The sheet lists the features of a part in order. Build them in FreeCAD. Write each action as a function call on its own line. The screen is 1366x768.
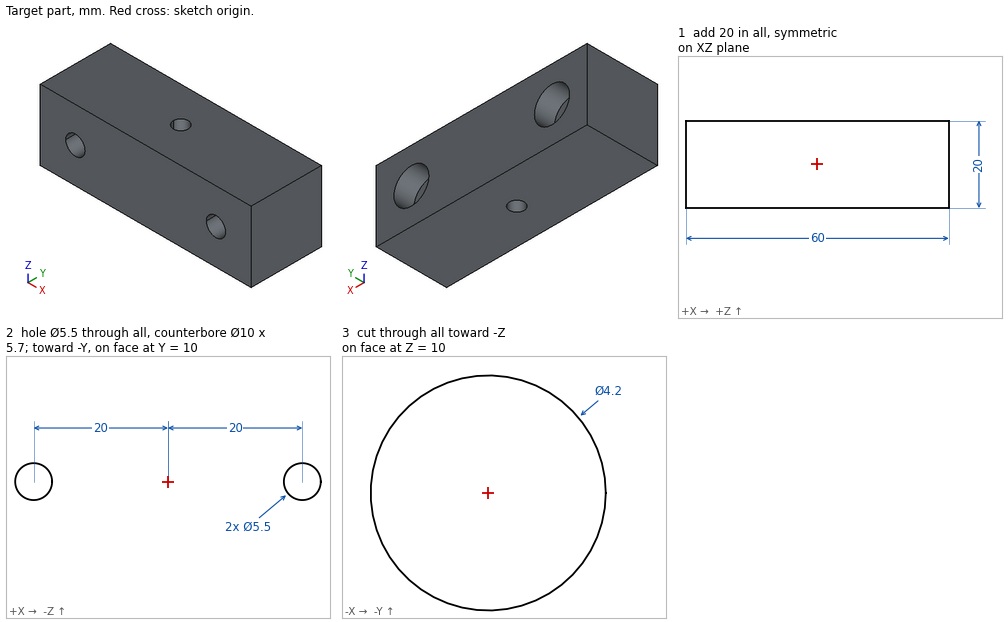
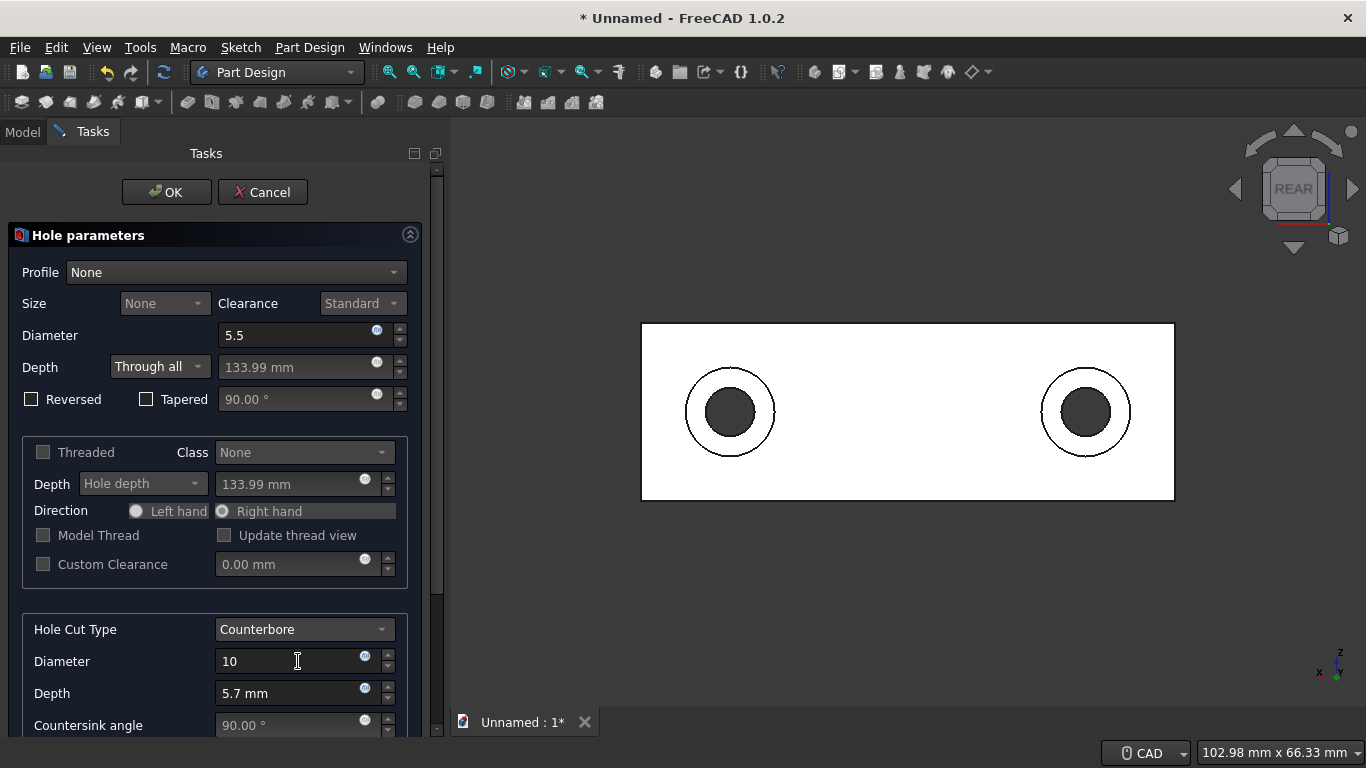
click(167, 192)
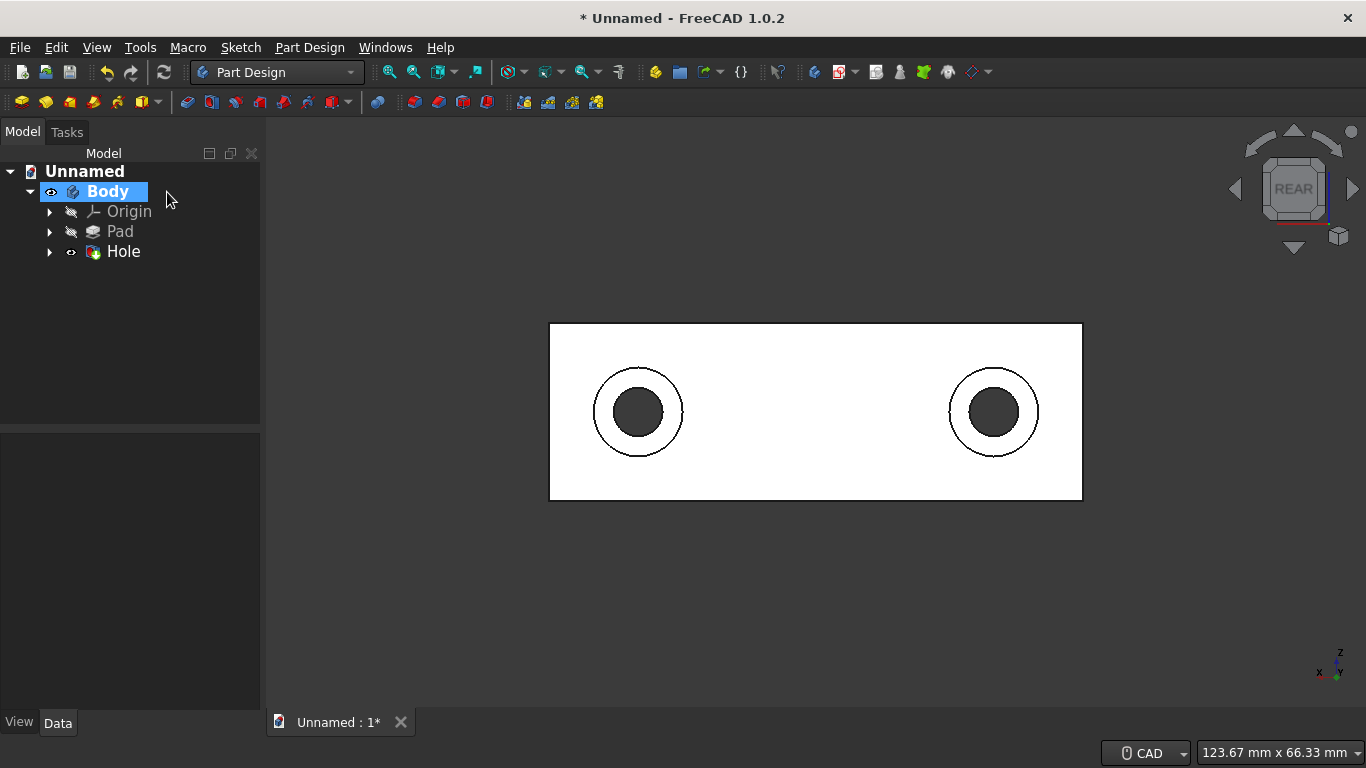
key(0)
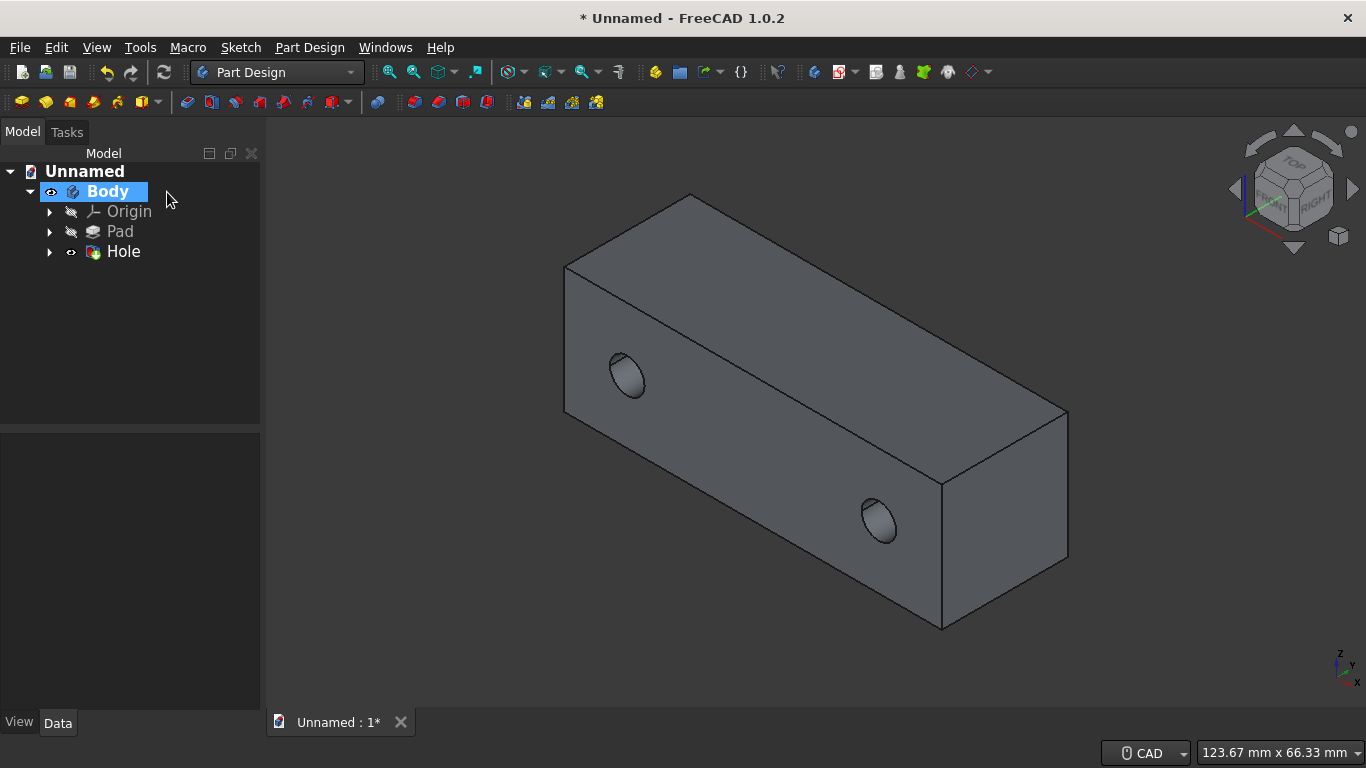
click(924, 401)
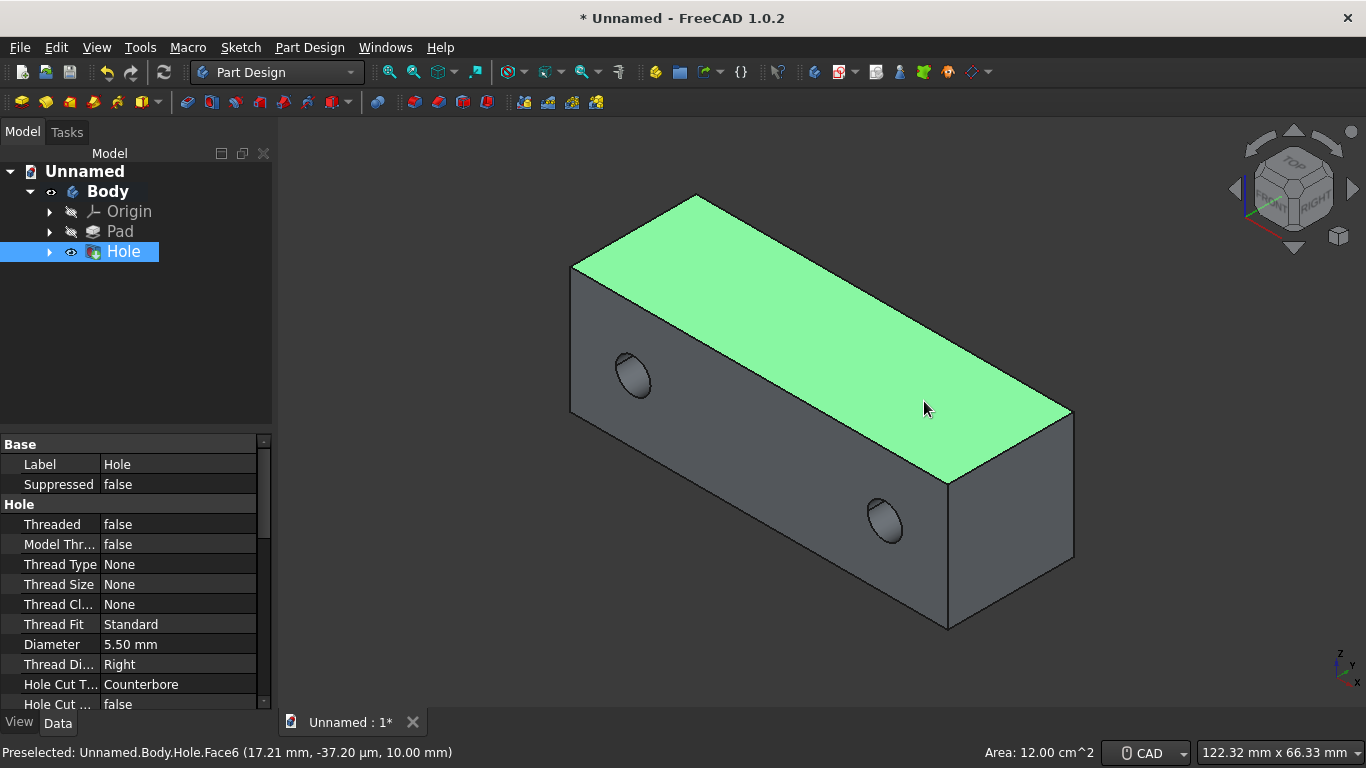
click(840, 72)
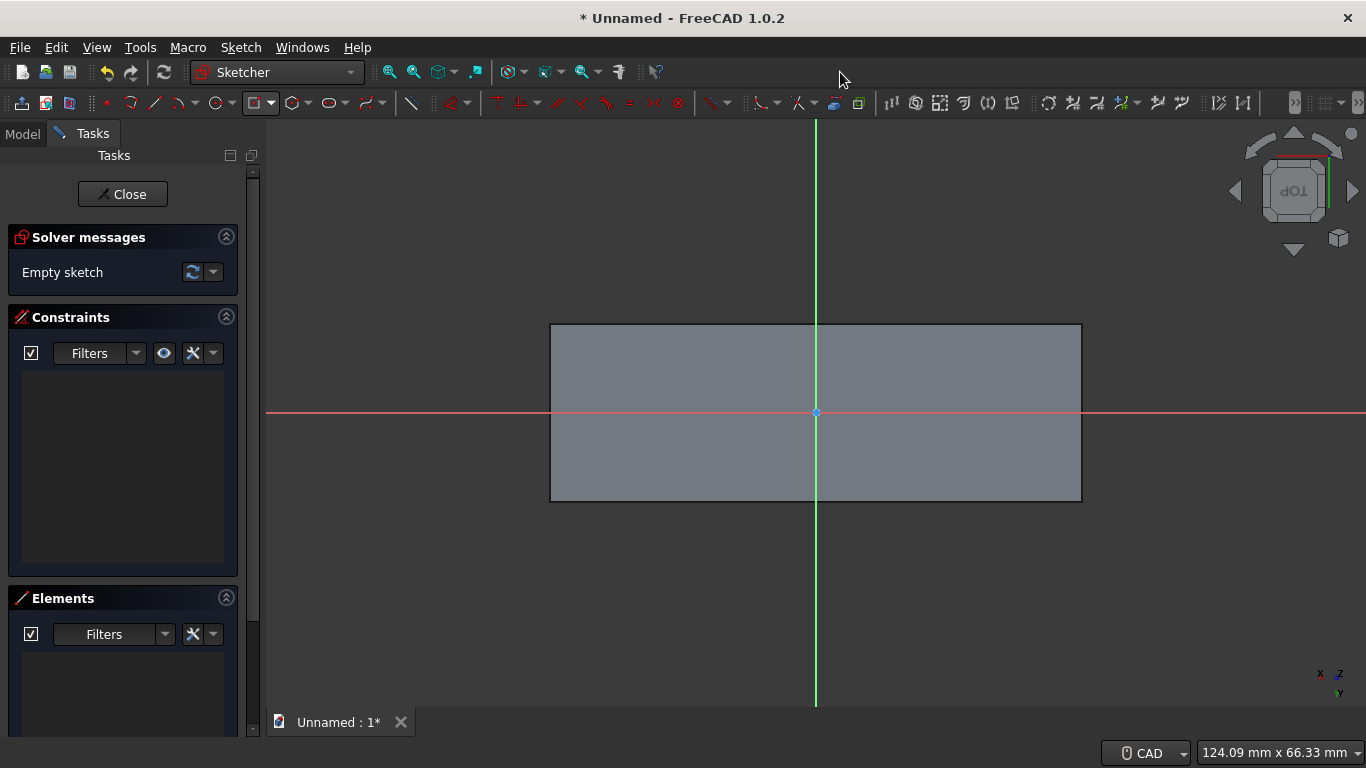
scroll(823, 413, up, 12)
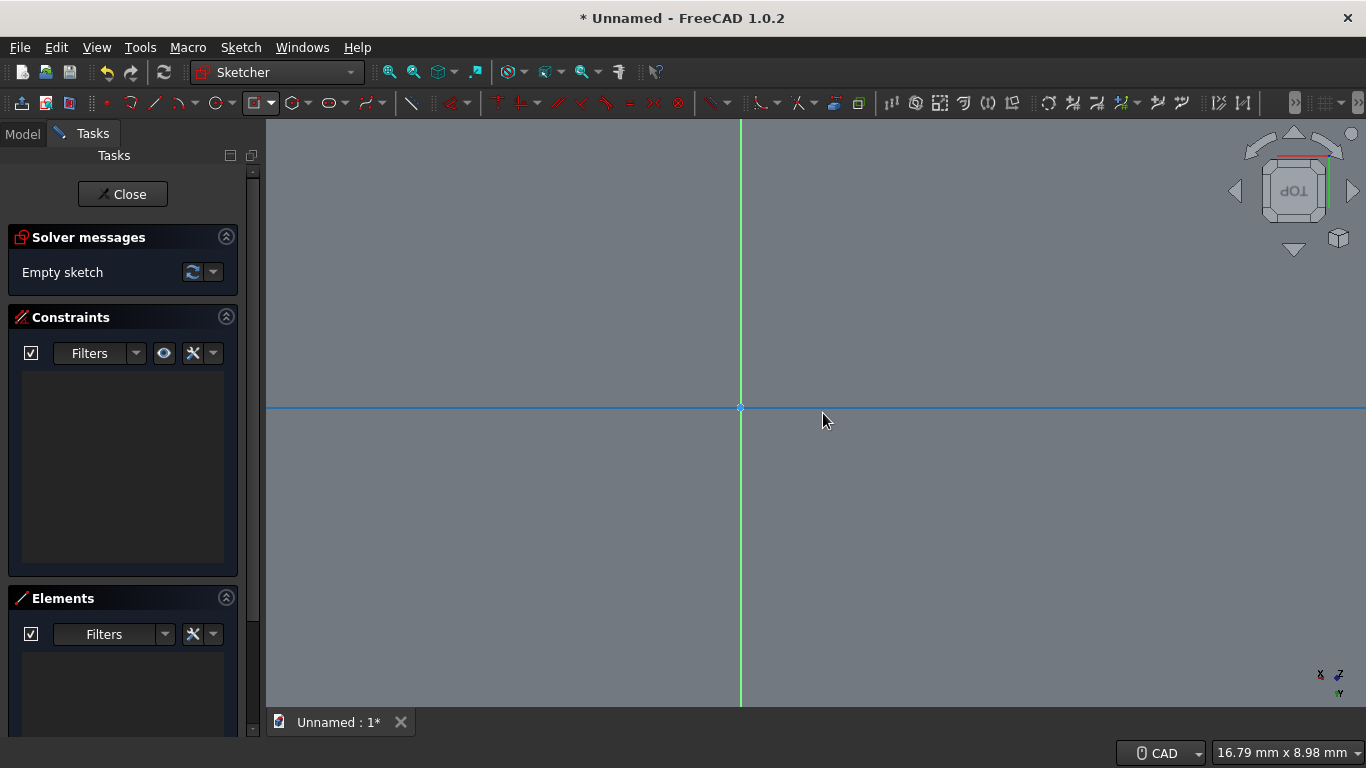
key(g)
key(c)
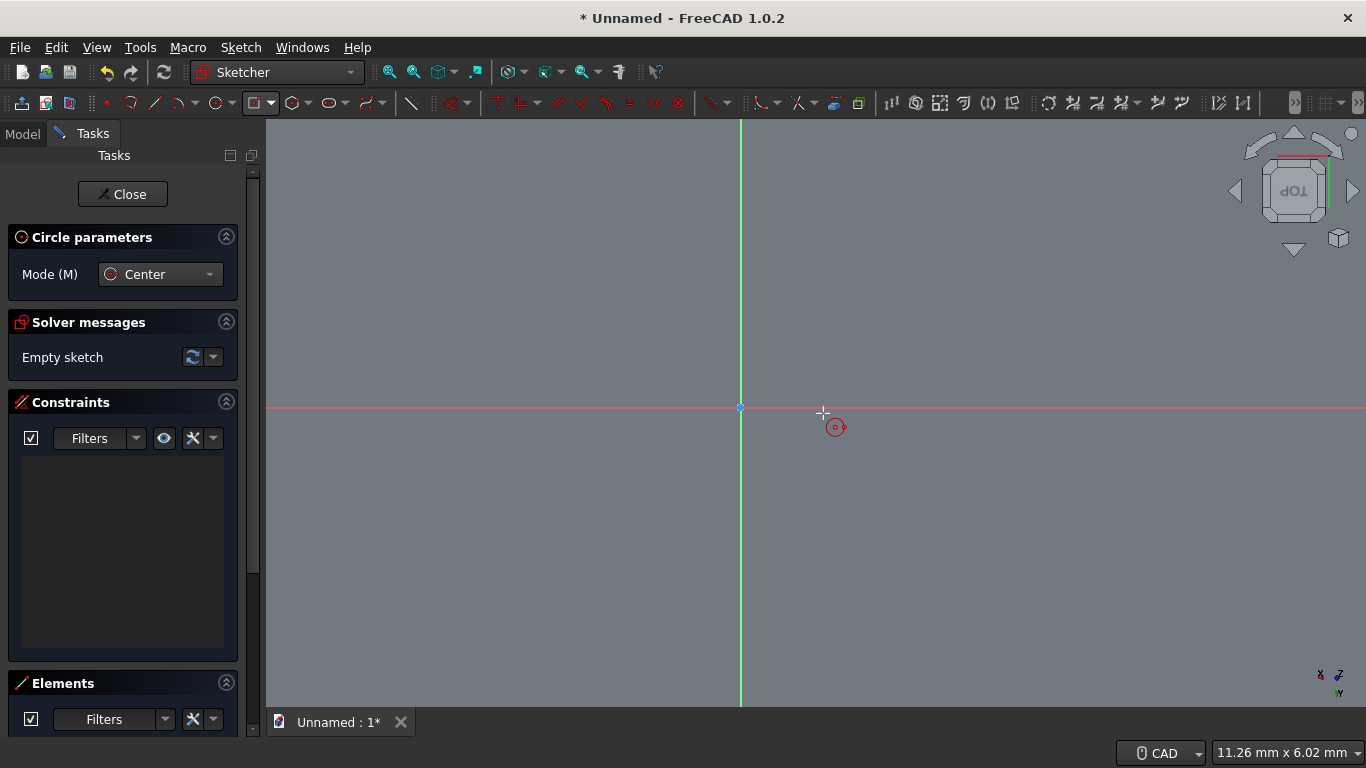
click(741, 408)
move(886, 263)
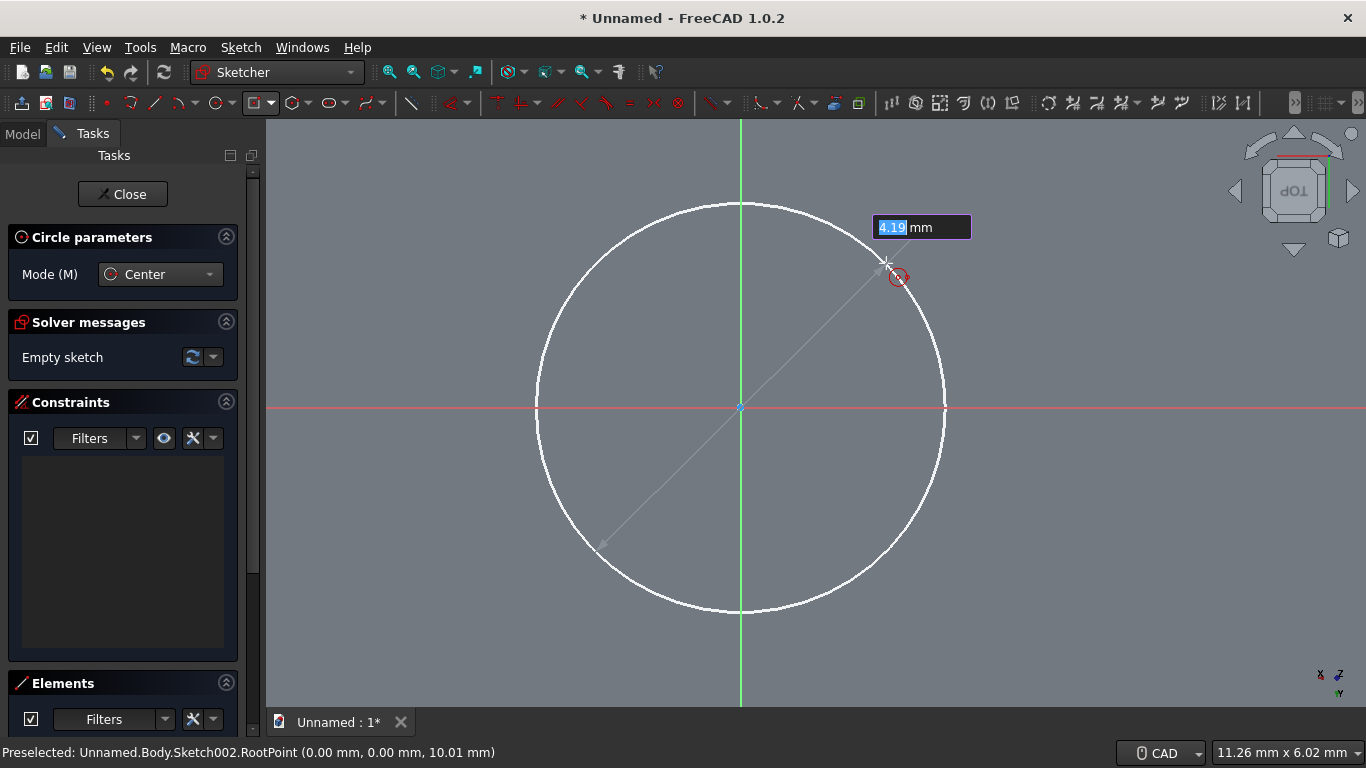
text(4.2)
key(Return)
key(Escape)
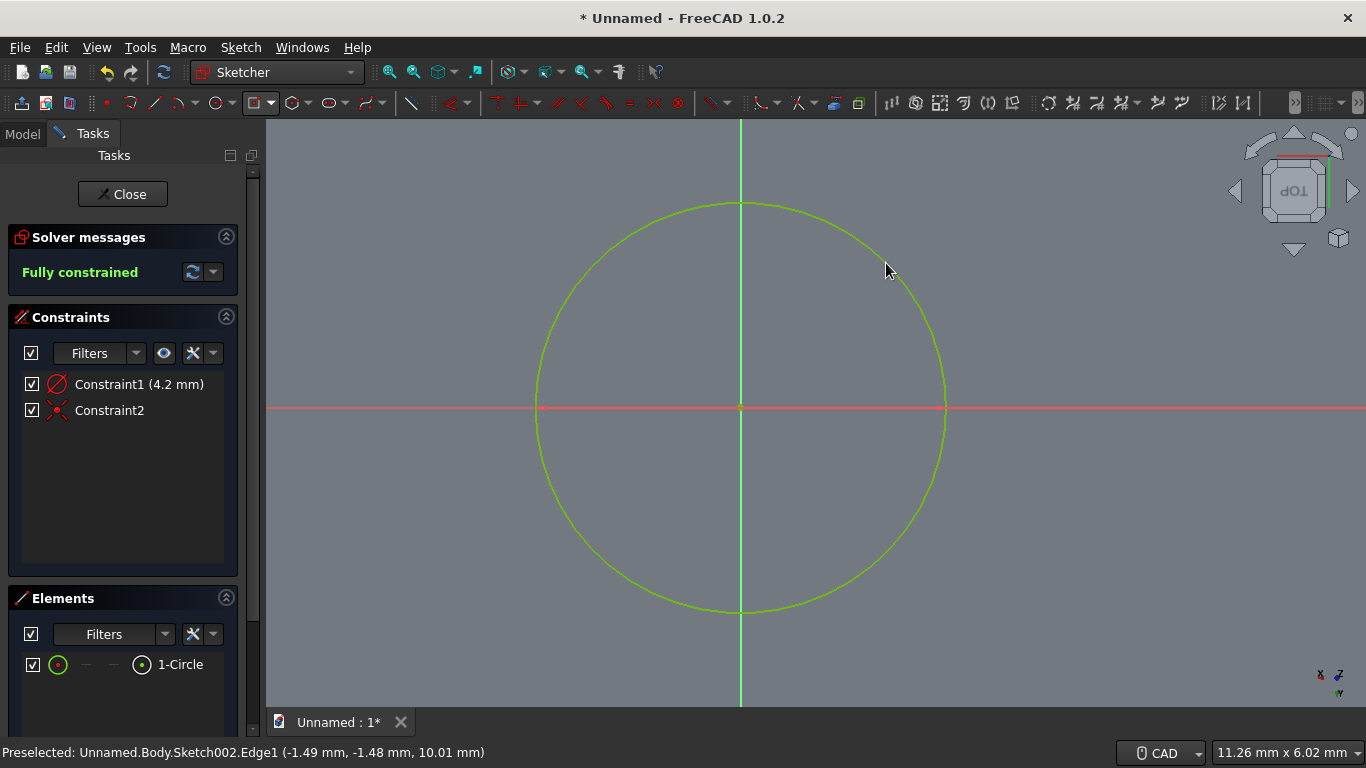
click(123, 194)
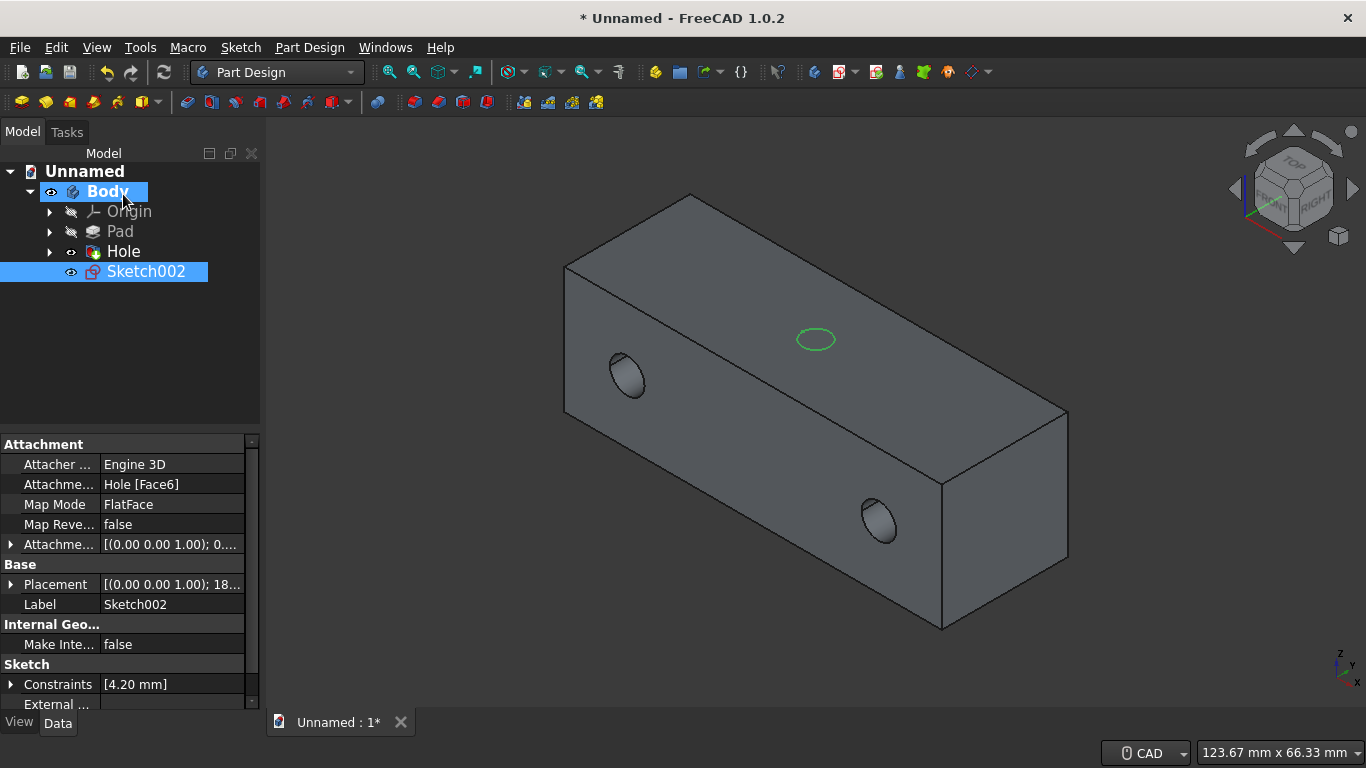
click(188, 102)